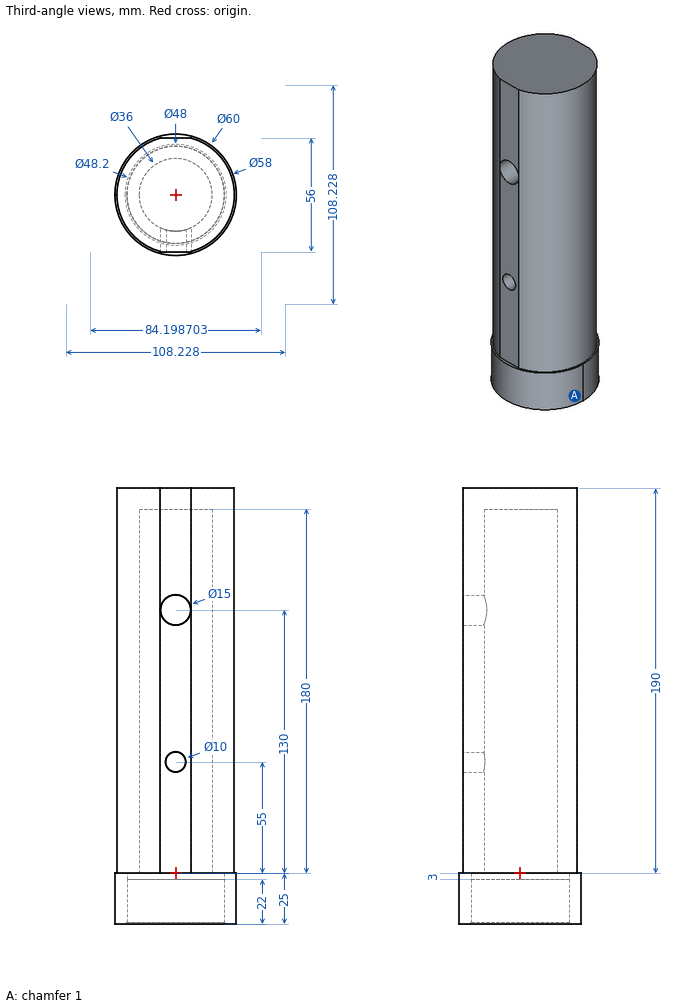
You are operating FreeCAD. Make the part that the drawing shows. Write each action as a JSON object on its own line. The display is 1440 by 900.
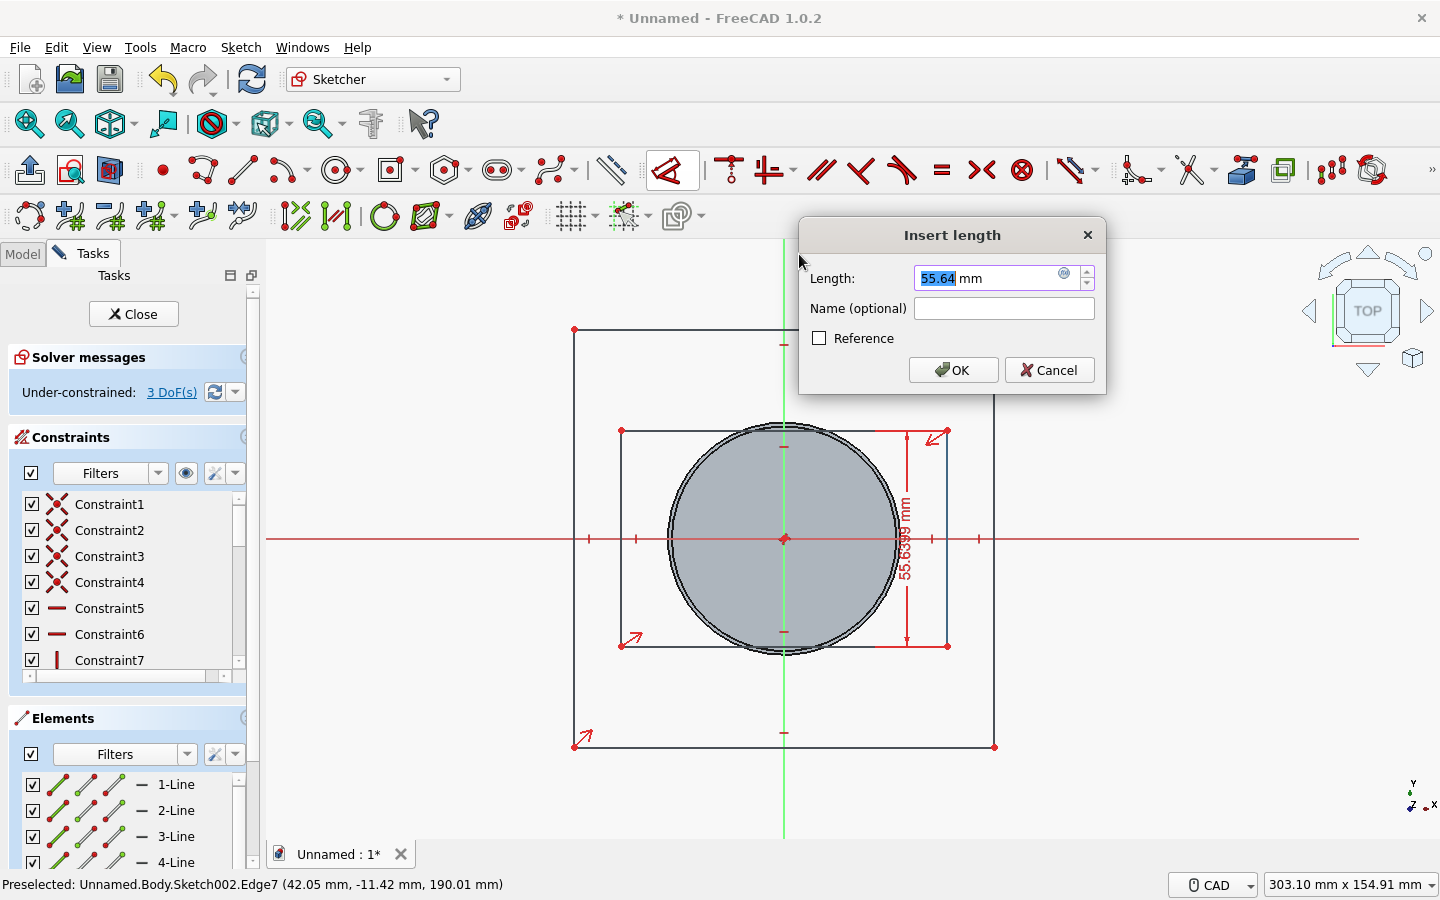
{"action": "type", "text": "56"}
{"action": "key", "text": "Return"}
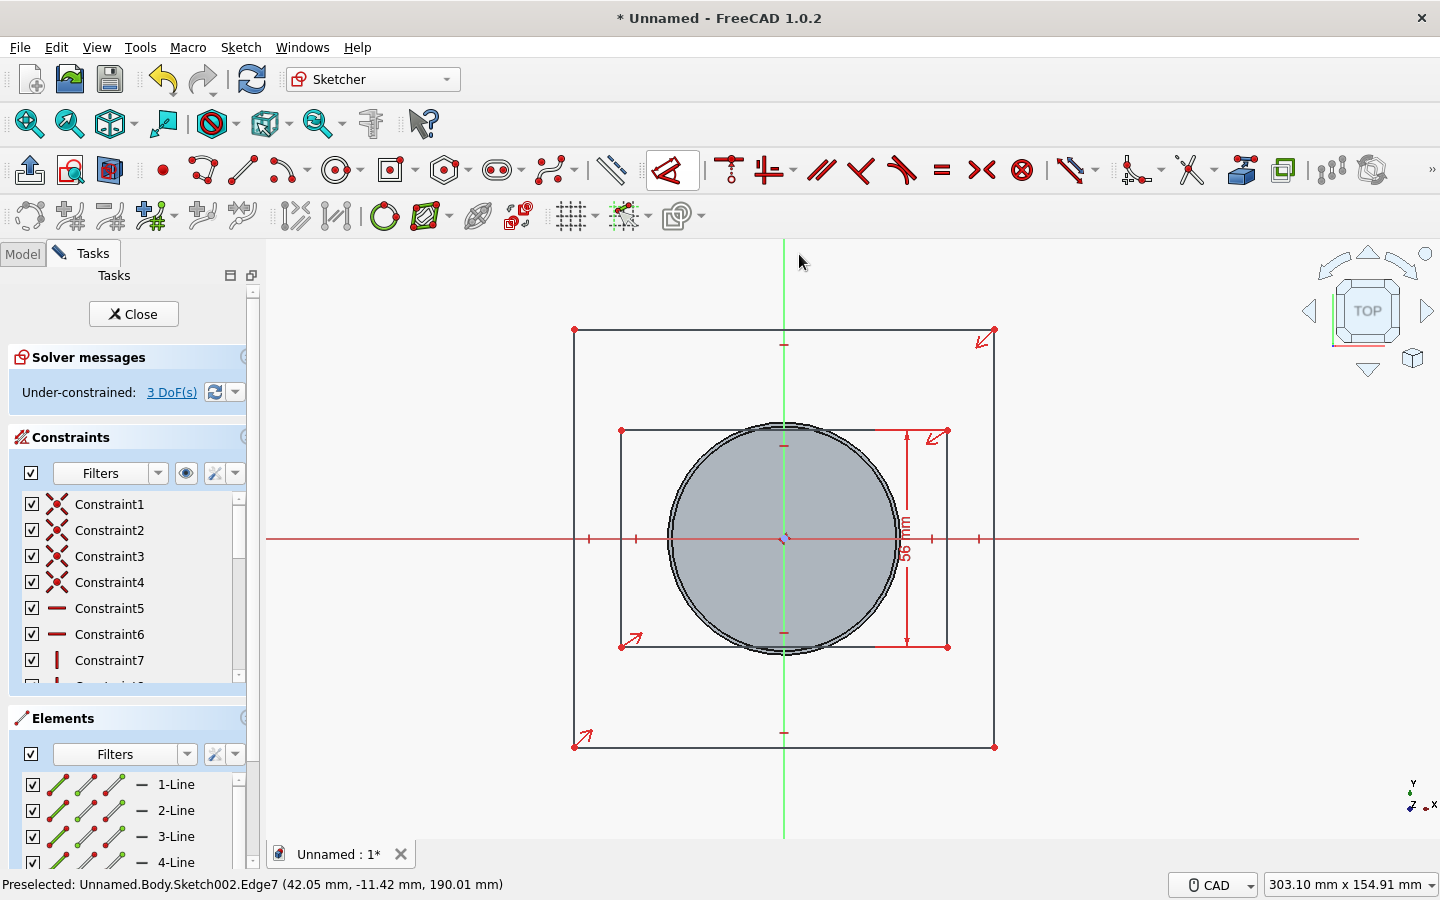
{"action": "left_click", "coordinate": [700, 748]}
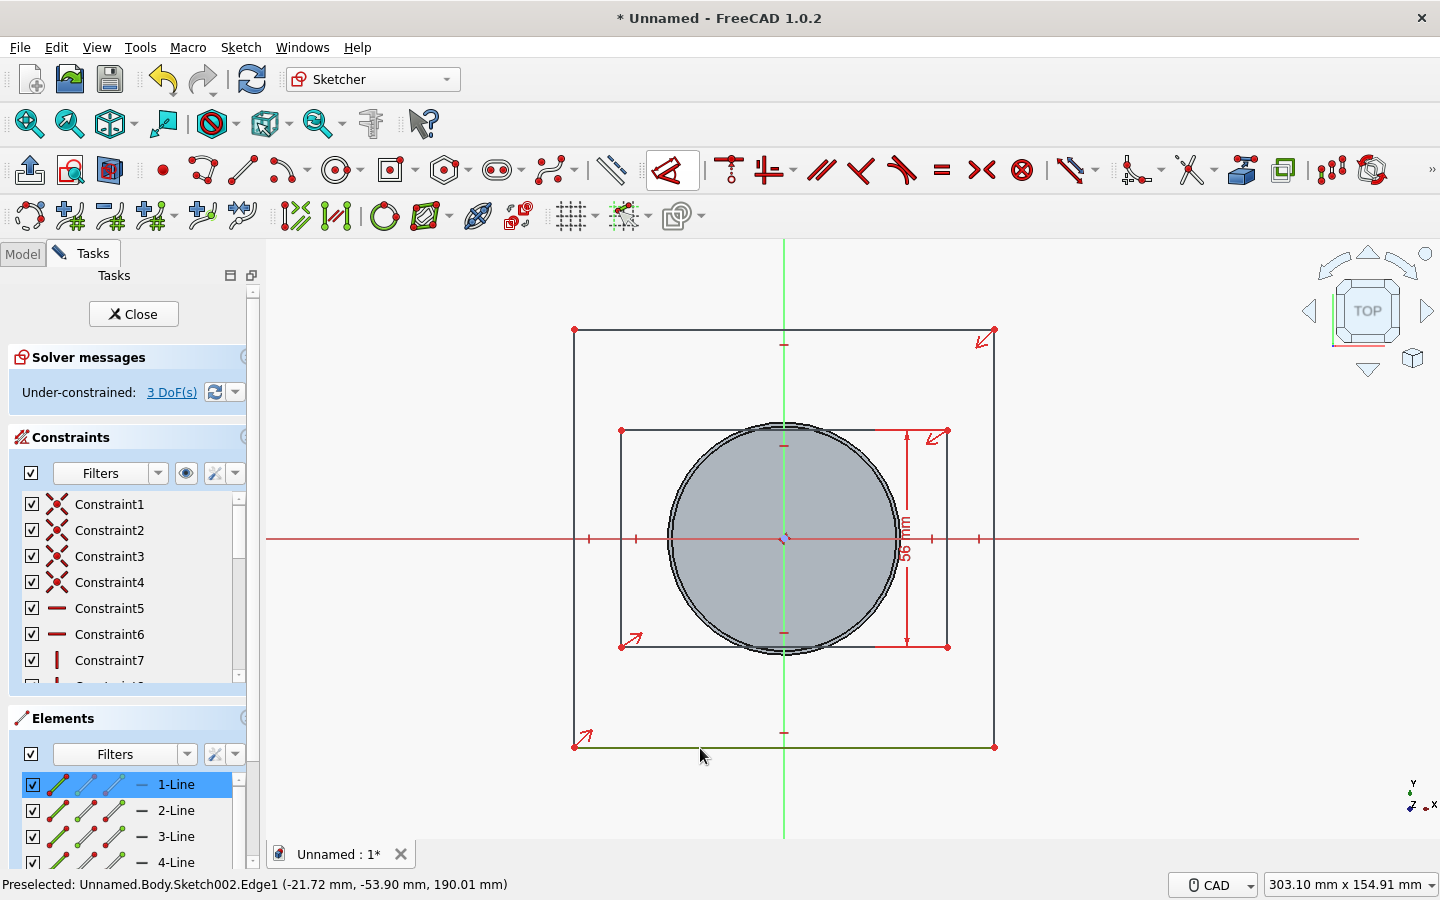
{"action": "left_click", "coordinate": [694, 170]}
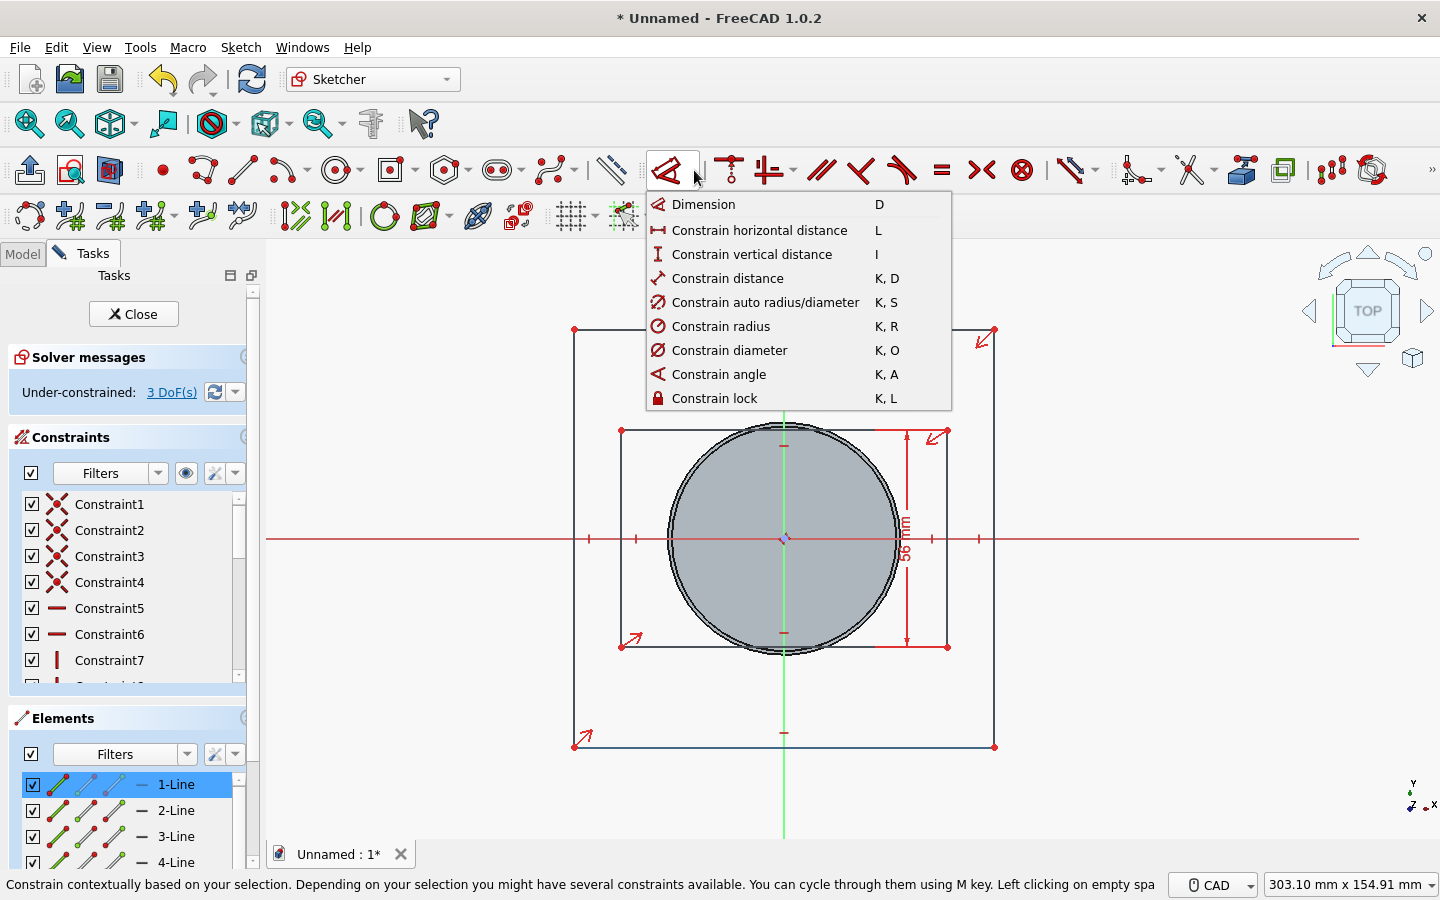
{"action": "left_click", "coordinate": [799, 230]}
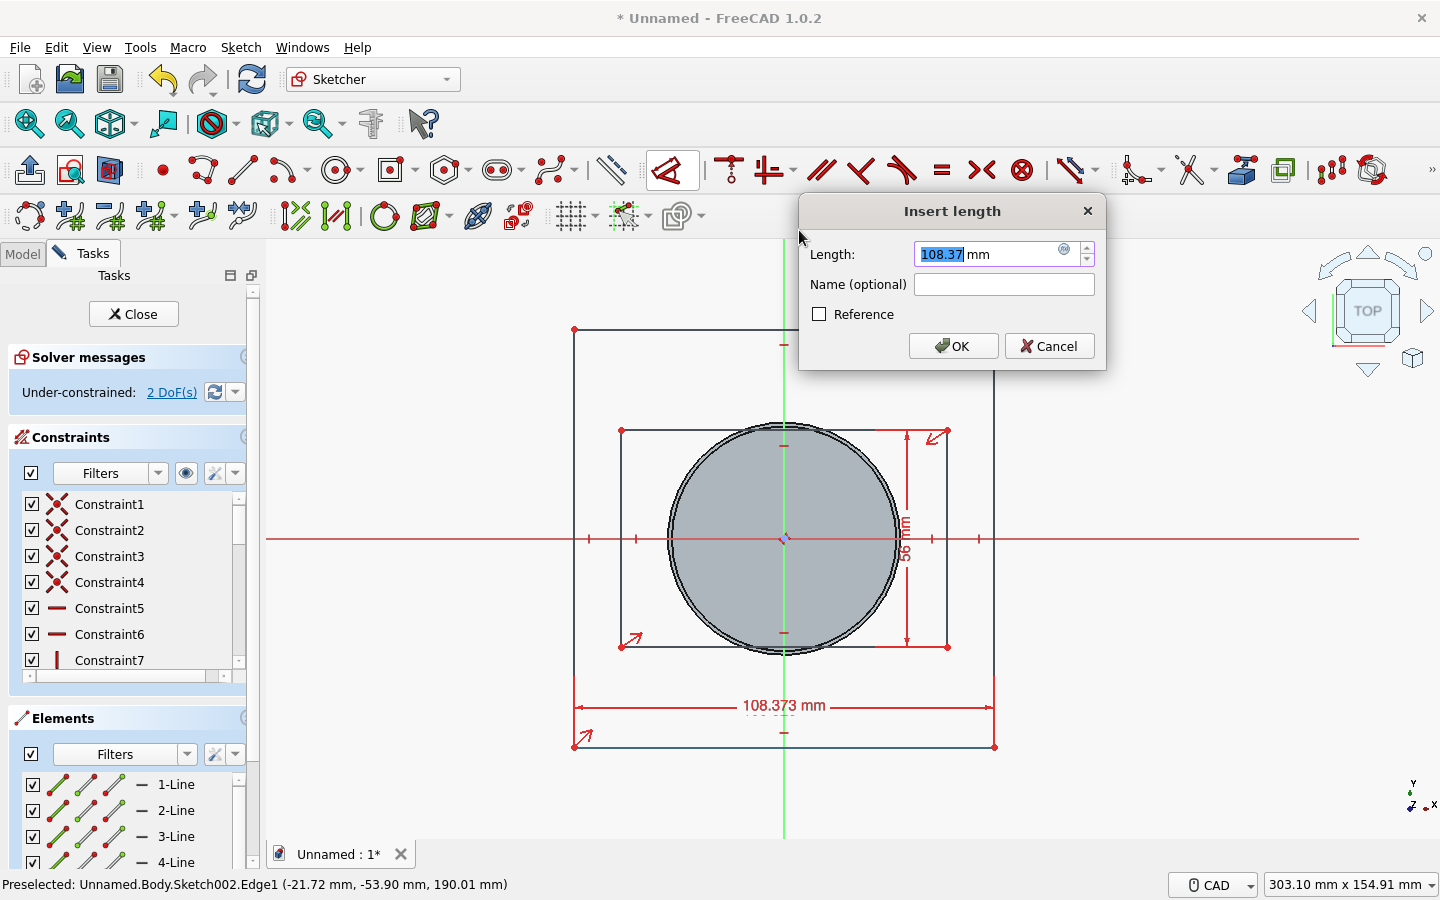
{"action": "type", "text": "108.228"}
{"action": "key", "text": "Return"}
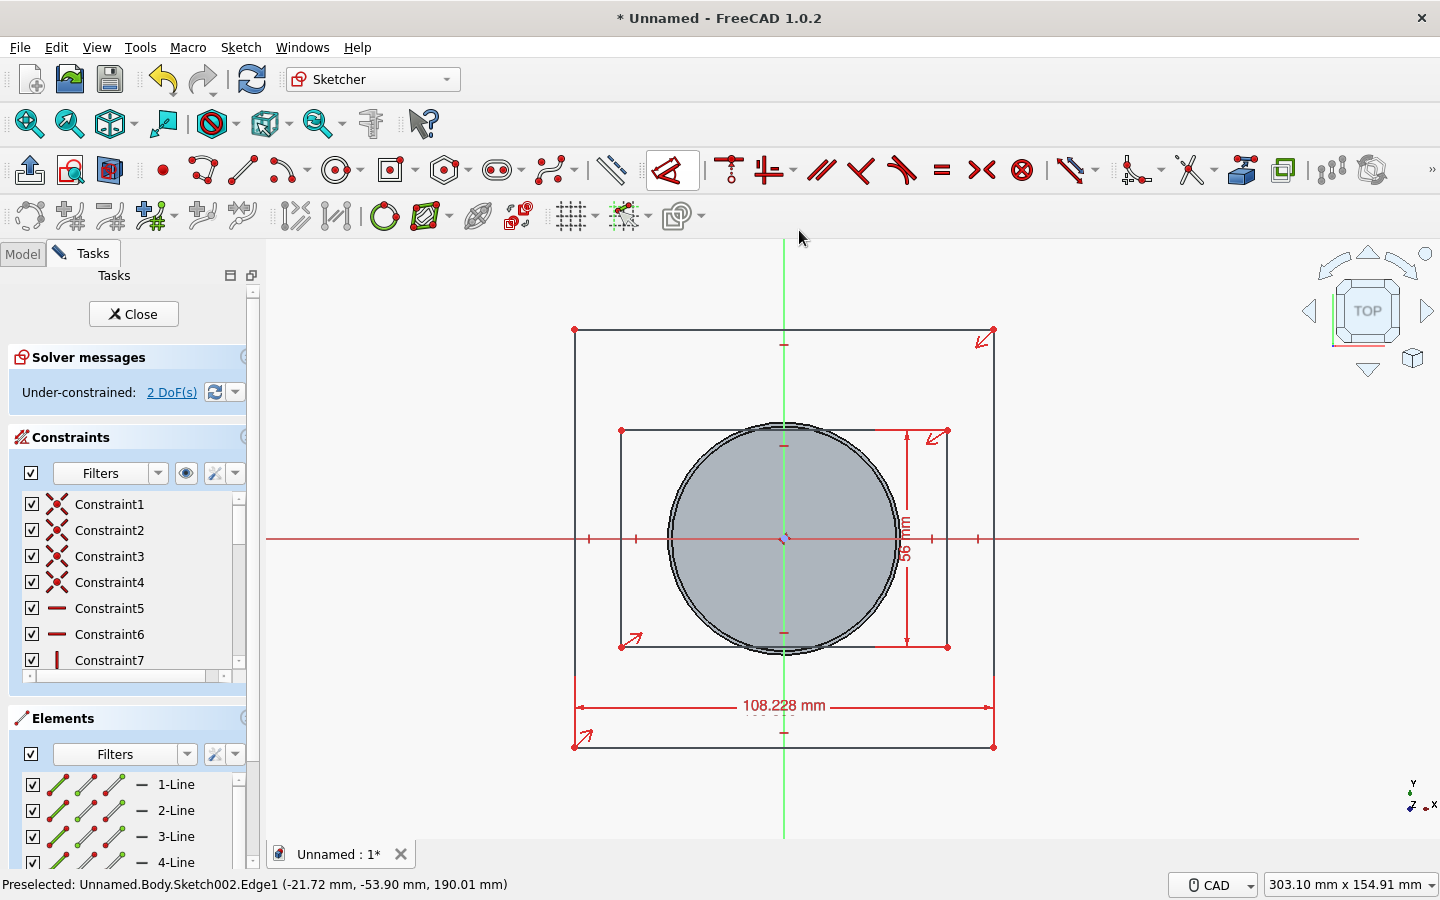
{"action": "left_click", "coordinate": [994, 622]}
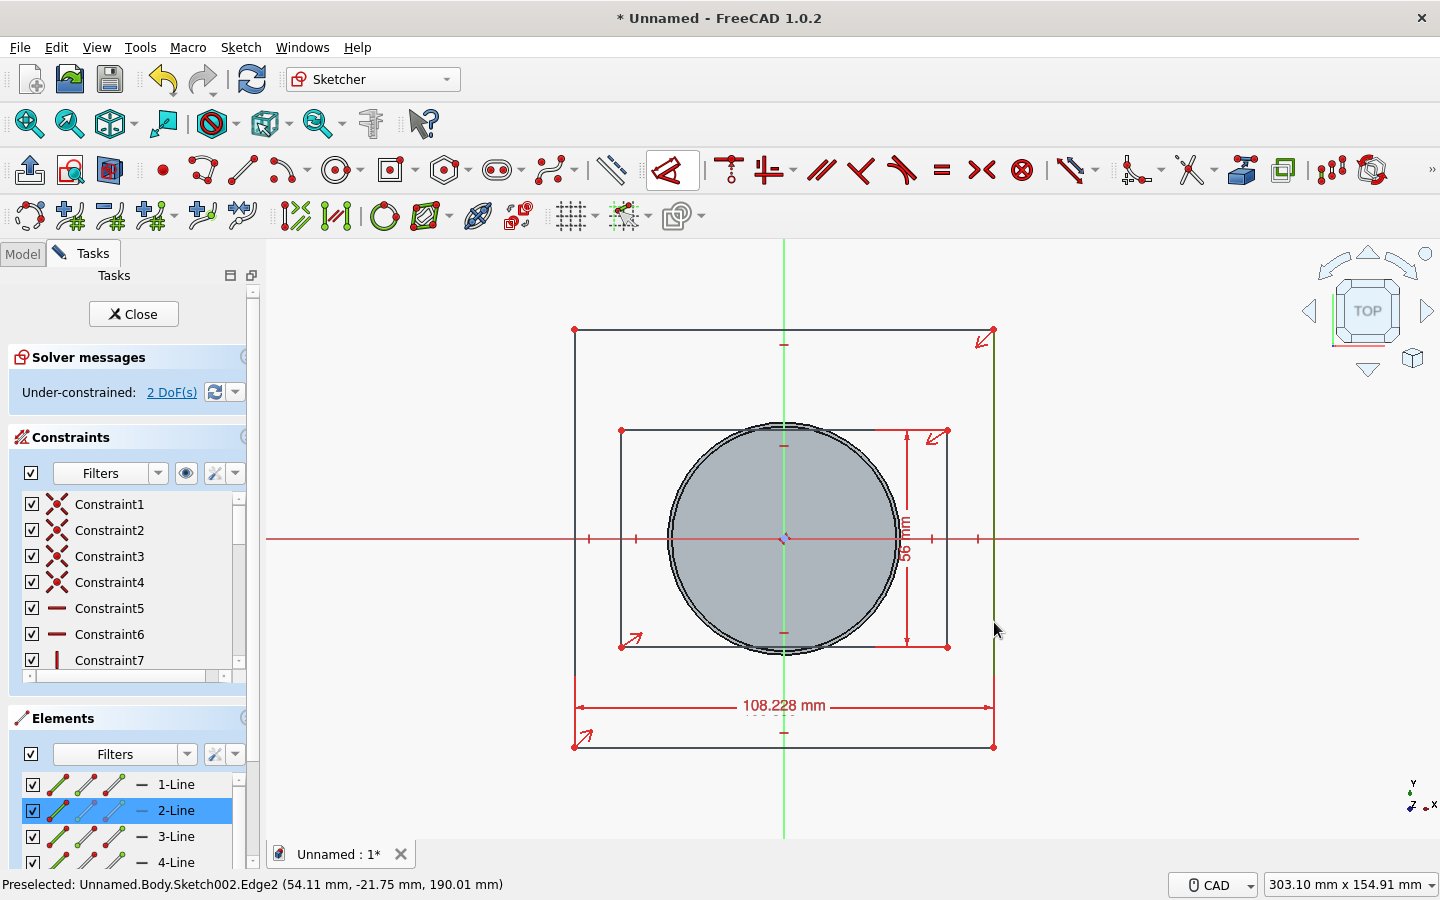
{"action": "left_click", "coordinate": [694, 170]}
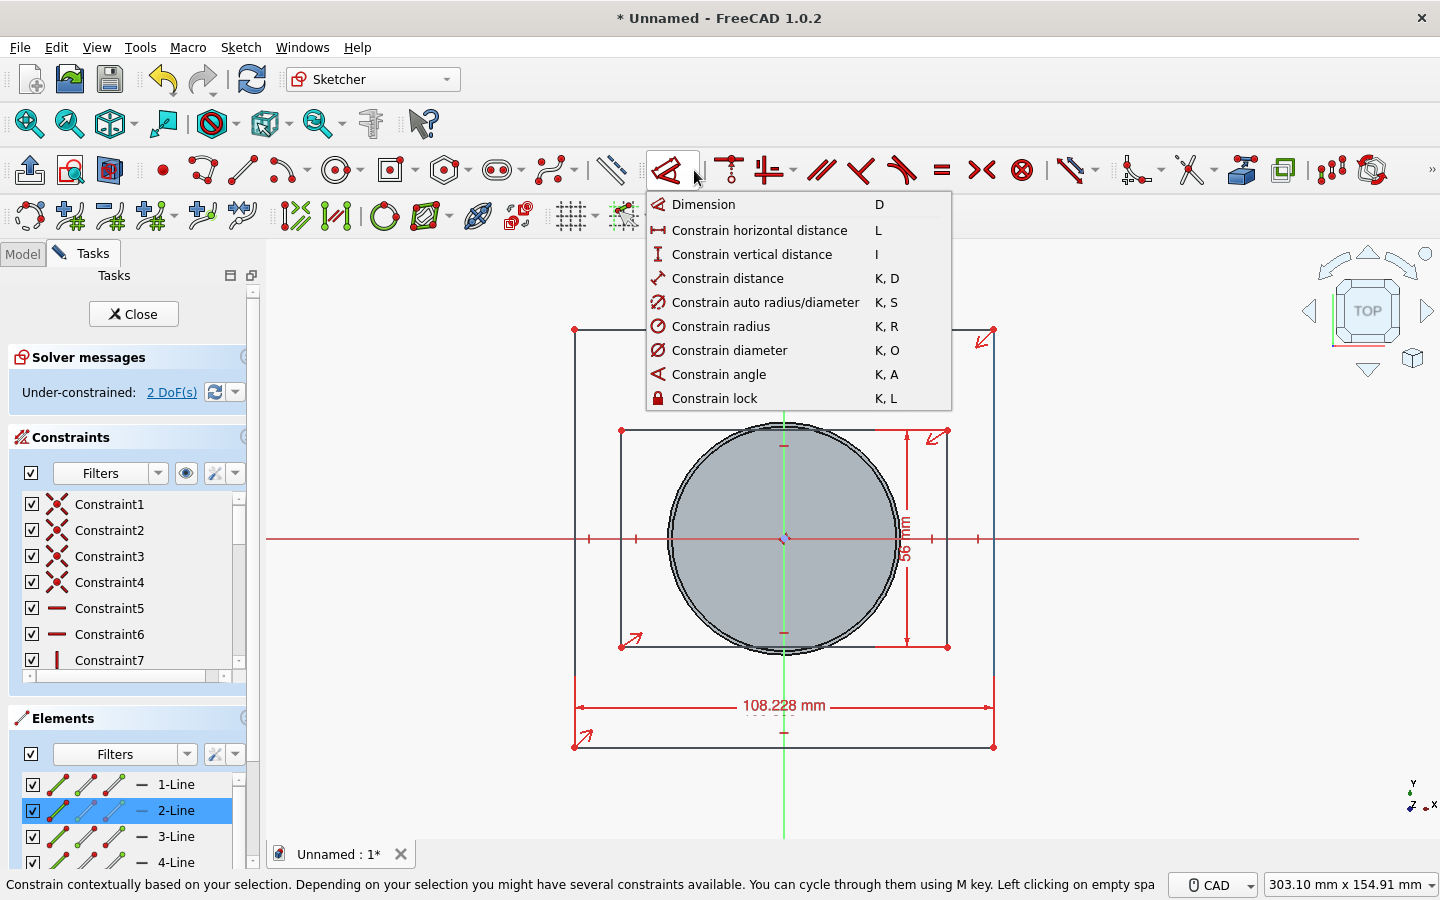
{"action": "left_click", "coordinate": [799, 254]}